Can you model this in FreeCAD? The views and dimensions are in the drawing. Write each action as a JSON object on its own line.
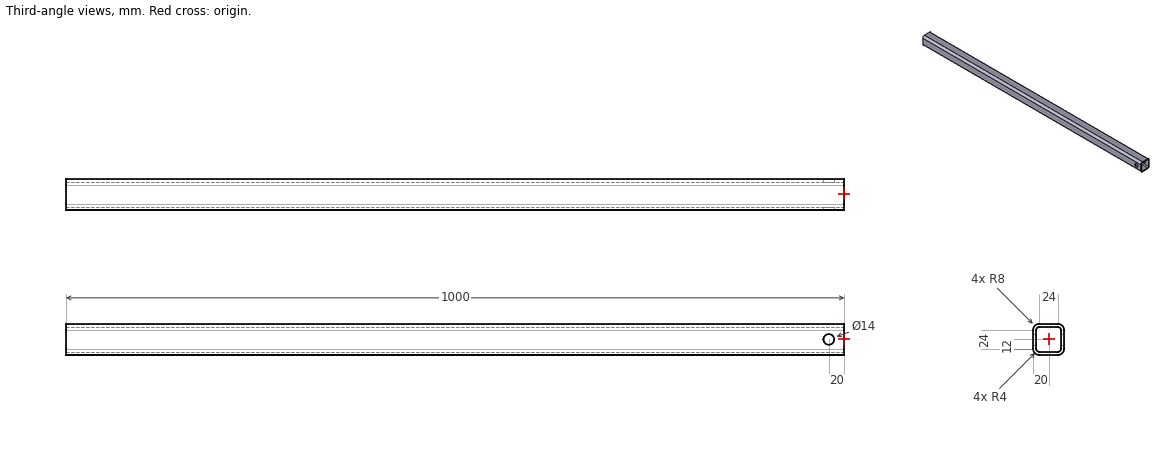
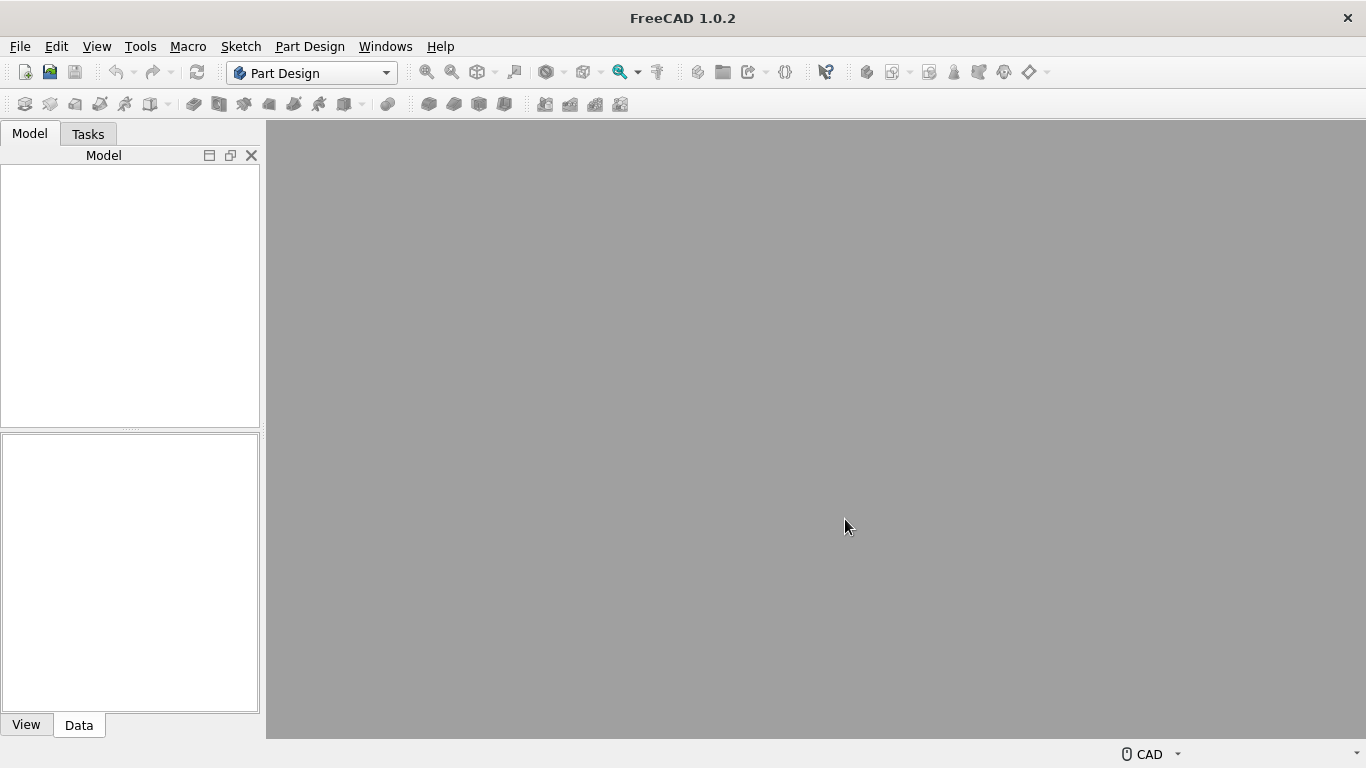
{"action": "left_click", "coordinate": [25, 72]}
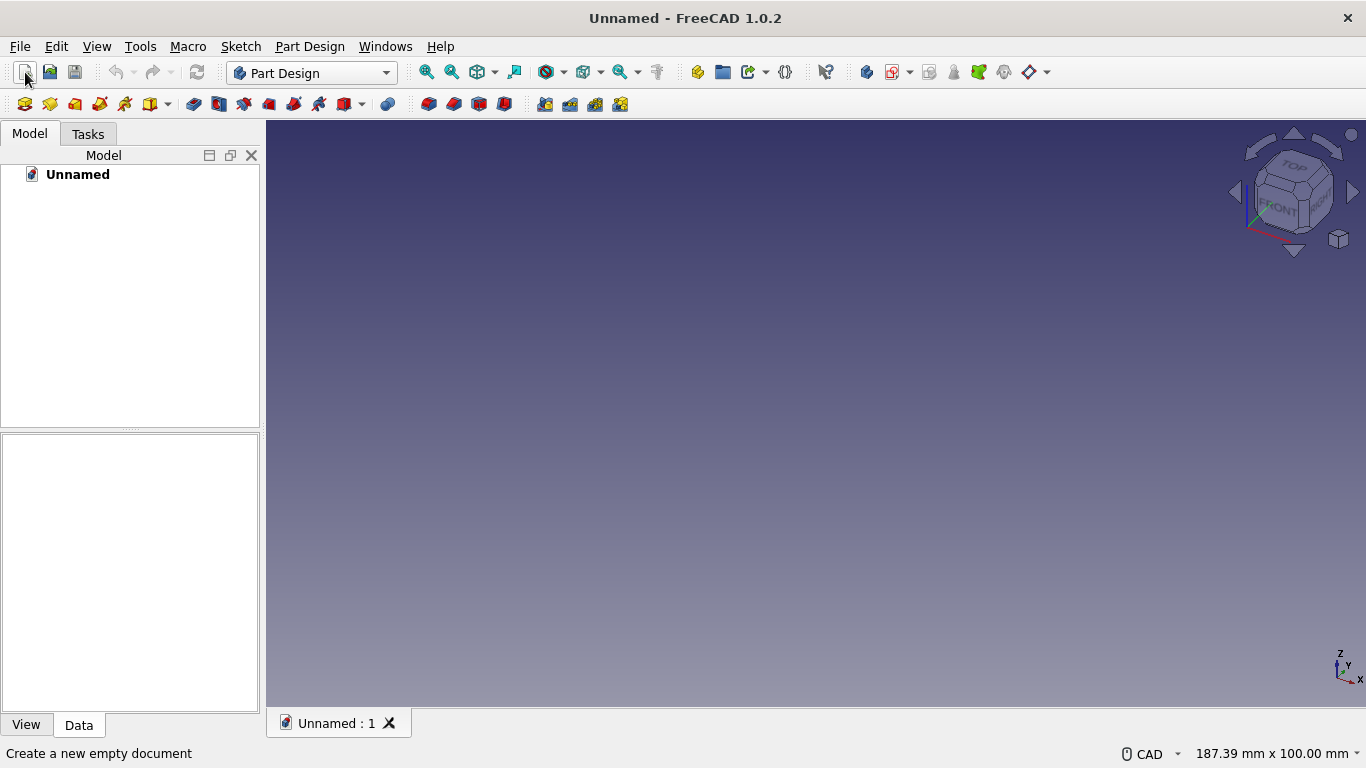
{"action": "left_click", "coordinate": [892, 72]}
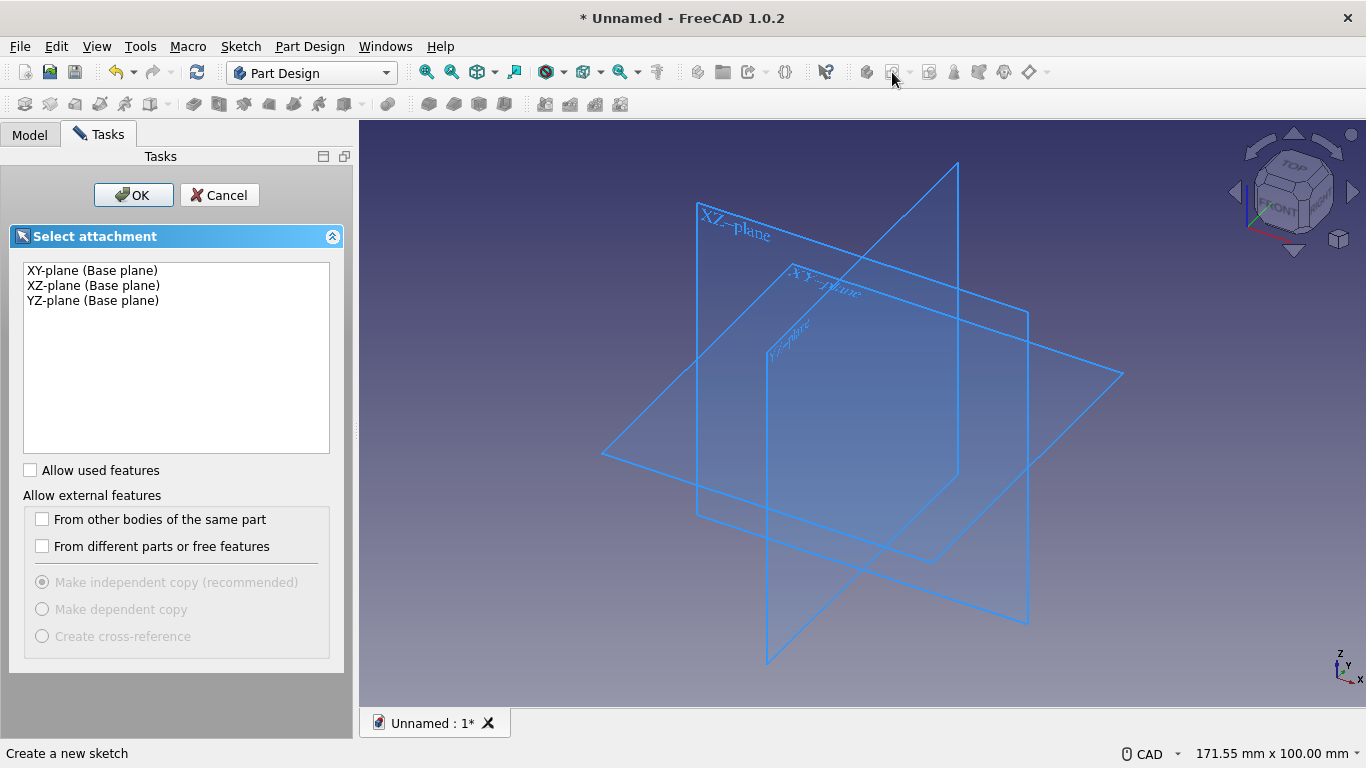
{"action": "left_click", "coordinate": [84, 300]}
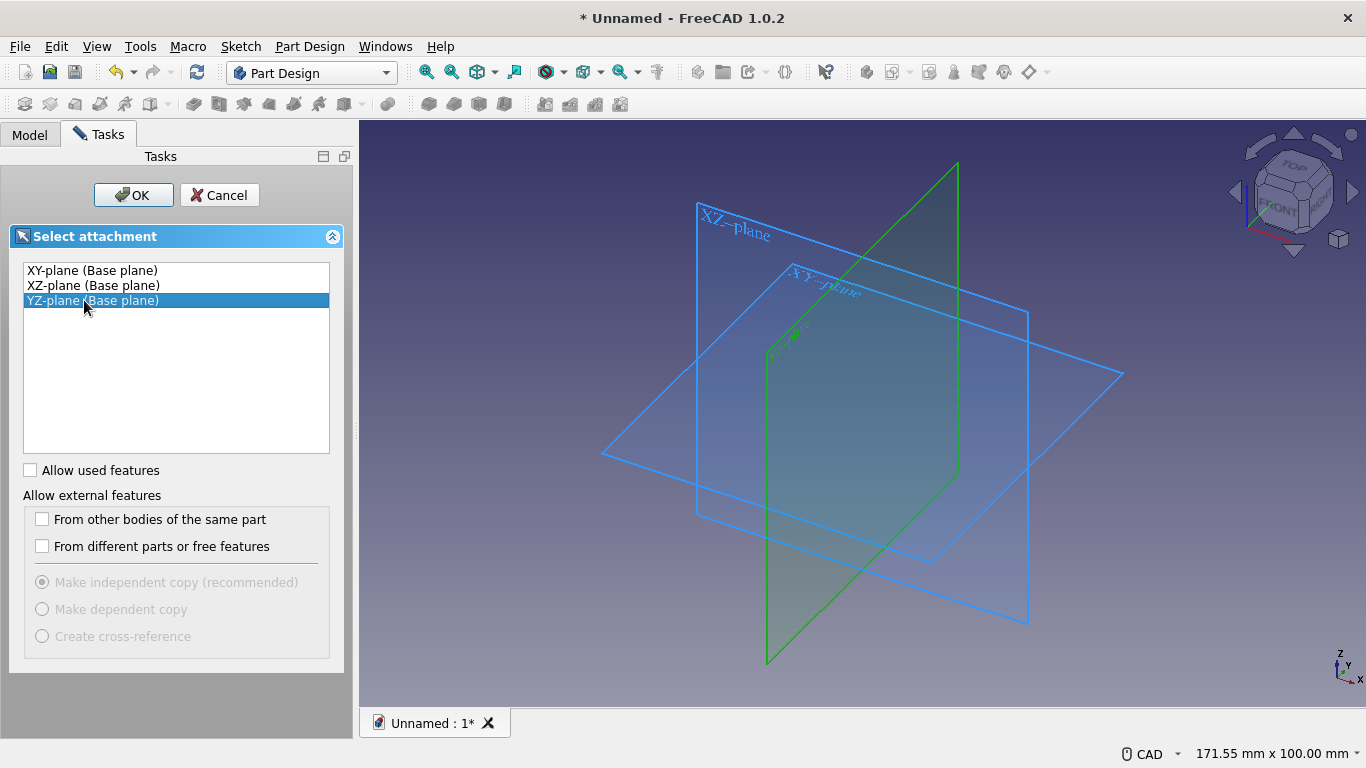
{"action": "left_click", "coordinate": [134, 195]}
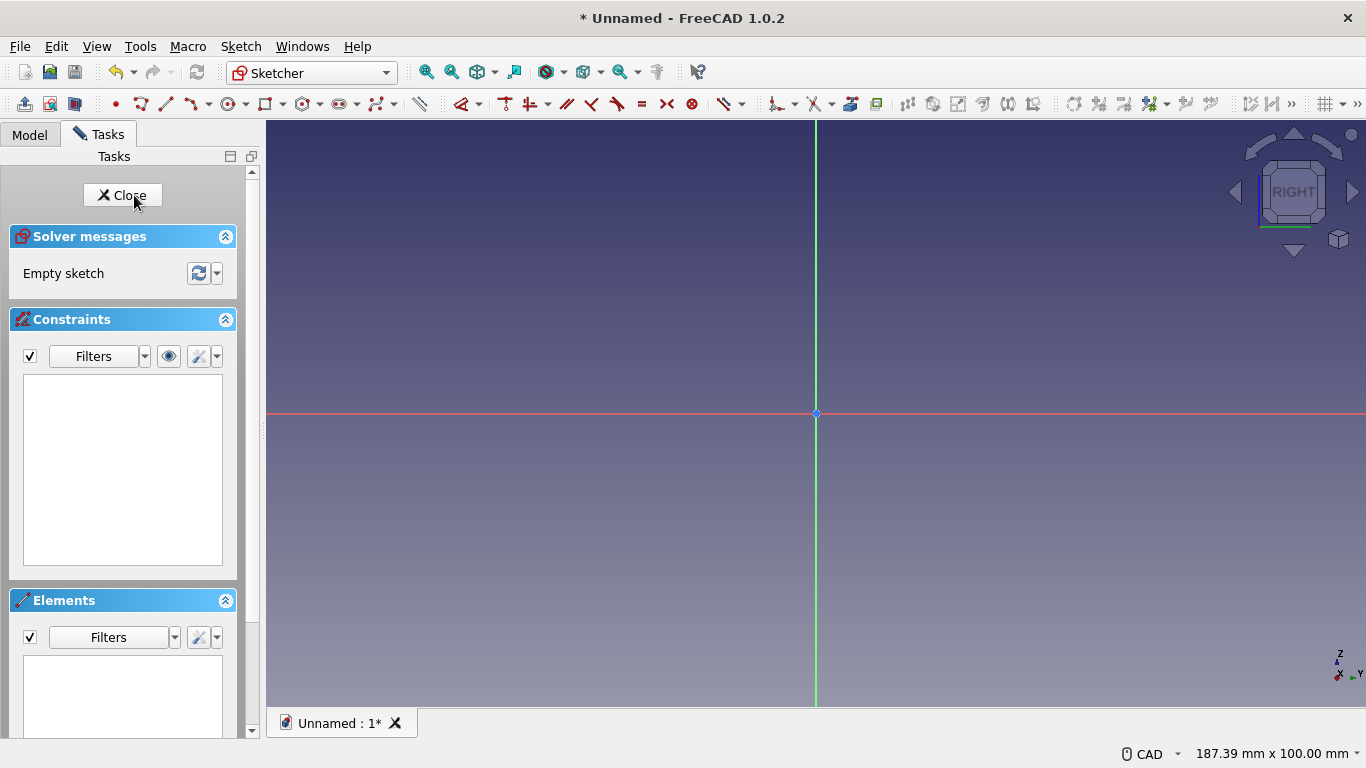
{"action": "scroll", "coordinate": [955, 413], "scroll_direction": "up", "scroll_amount": 2}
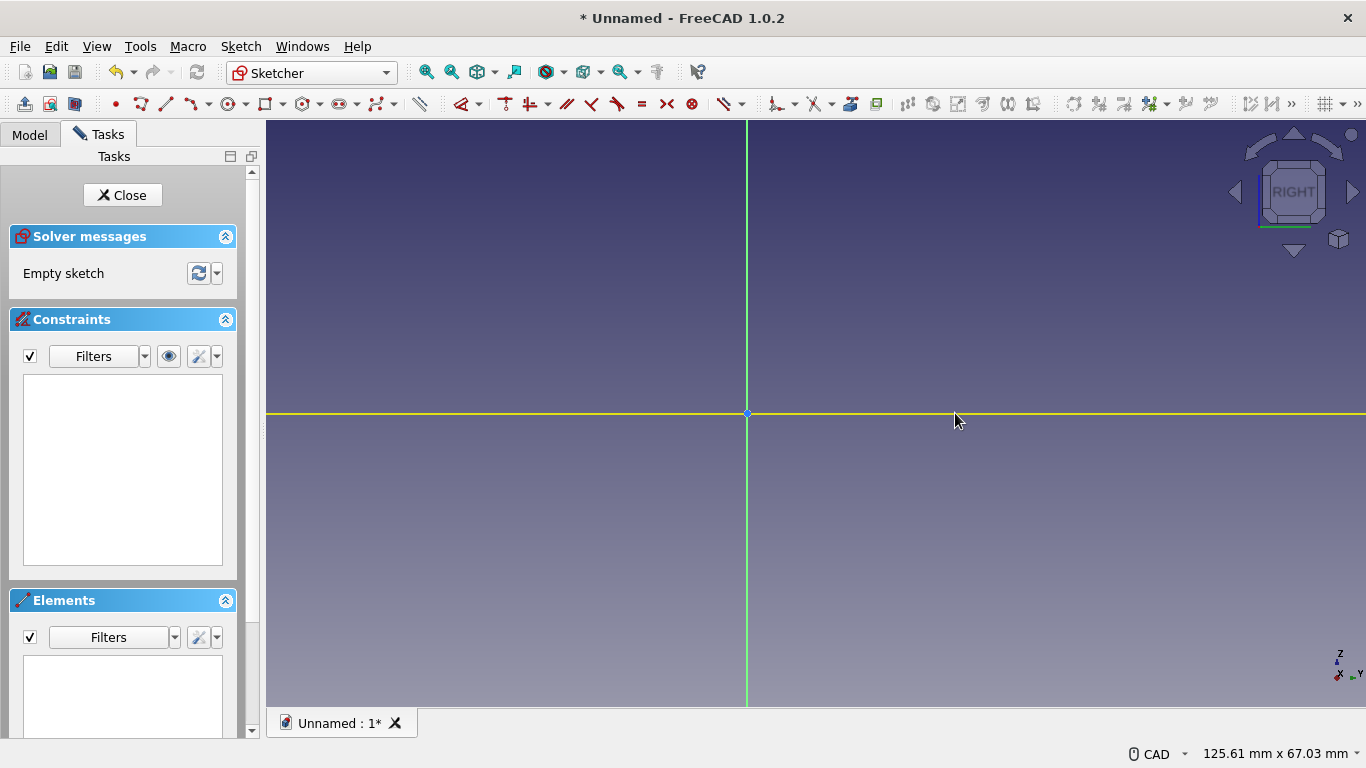
{"action": "left_click", "coordinate": [166, 104]}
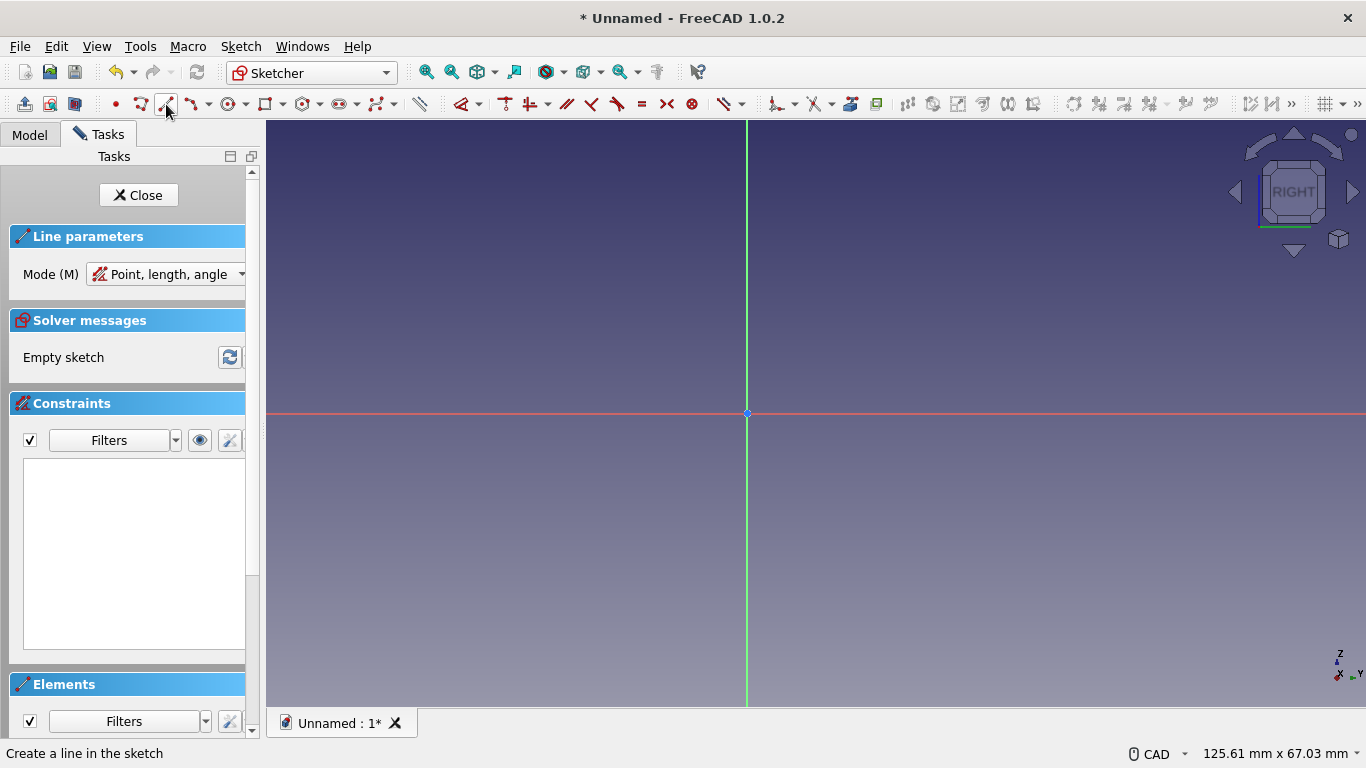
{"action": "left_click", "coordinate": [572, 519]}
{"action": "left_click", "coordinate": [572, 308]}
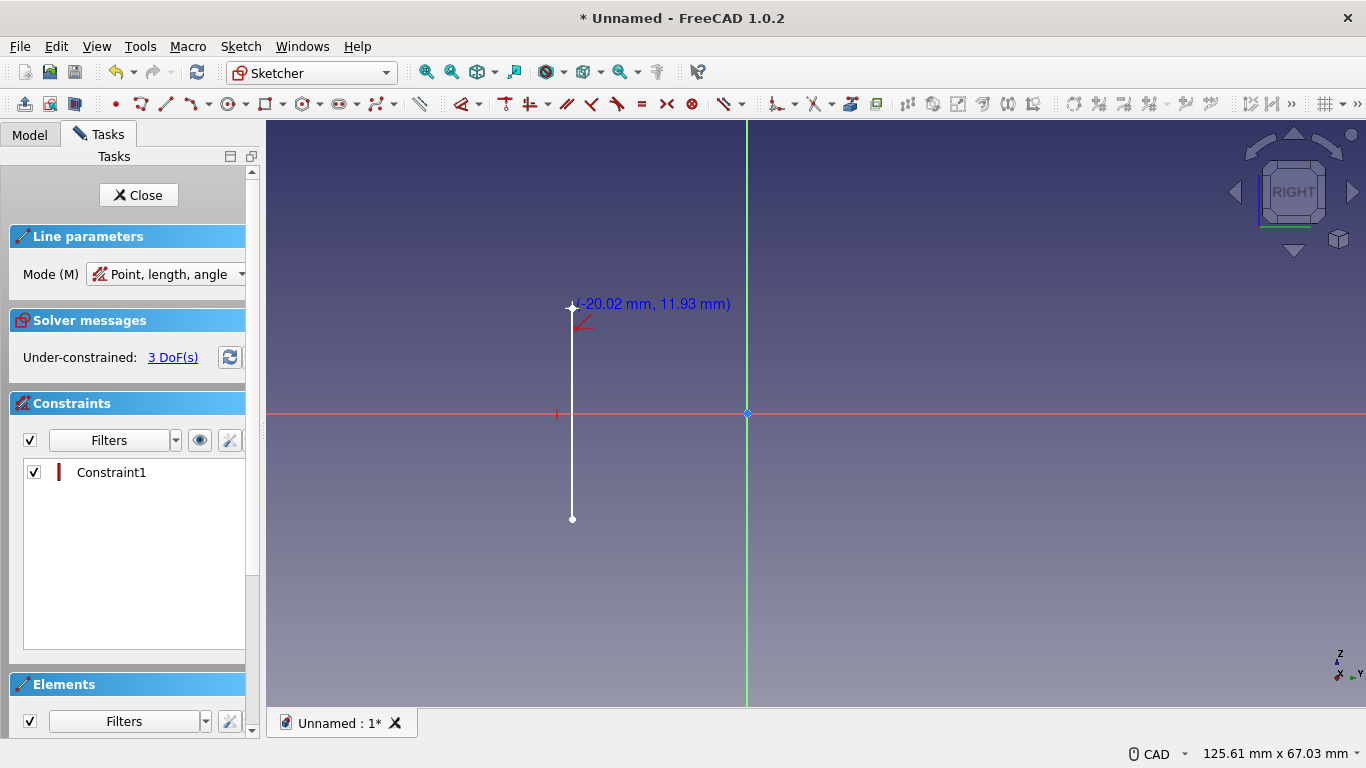
{"action": "left_click", "coordinate": [642, 238]}
{"action": "left_click", "coordinate": [852, 238]}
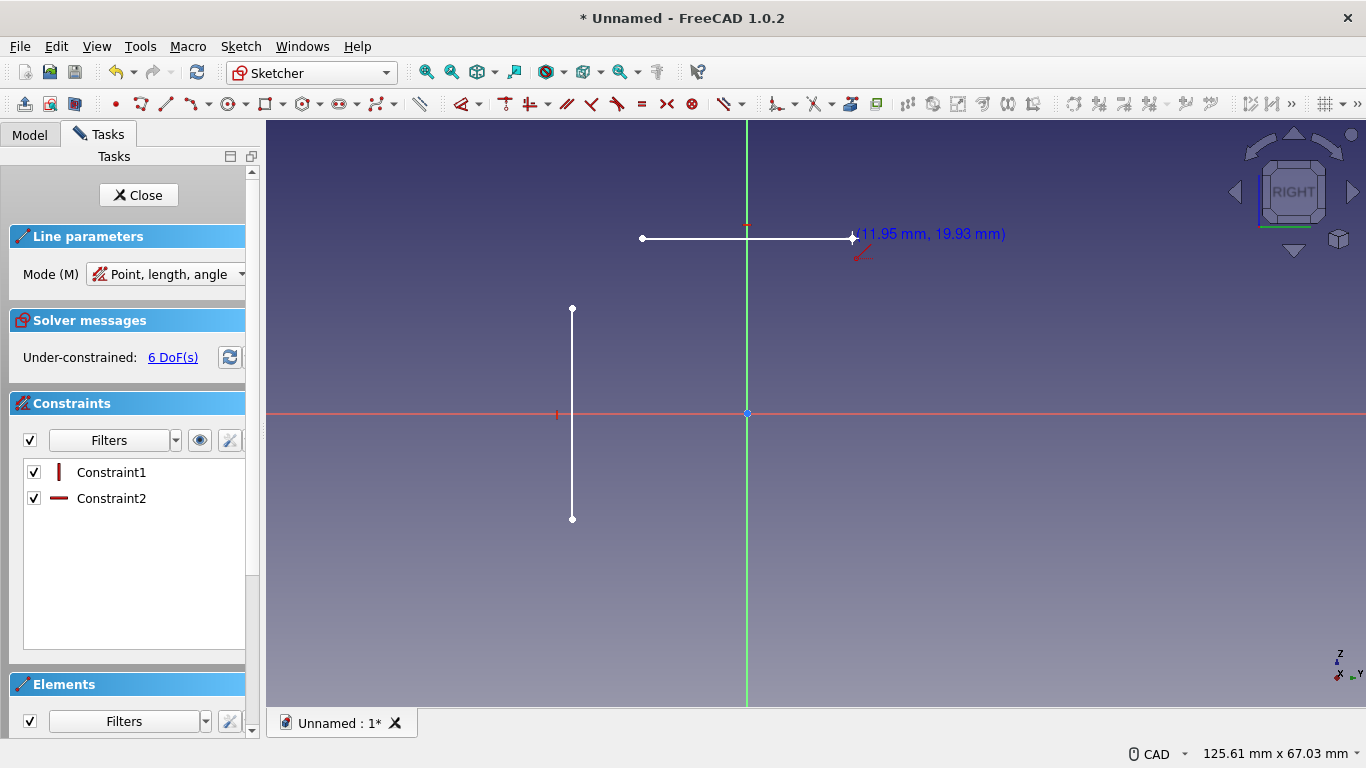
{"action": "left_click", "coordinate": [922, 308]}
{"action": "left_click", "coordinate": [922, 519]}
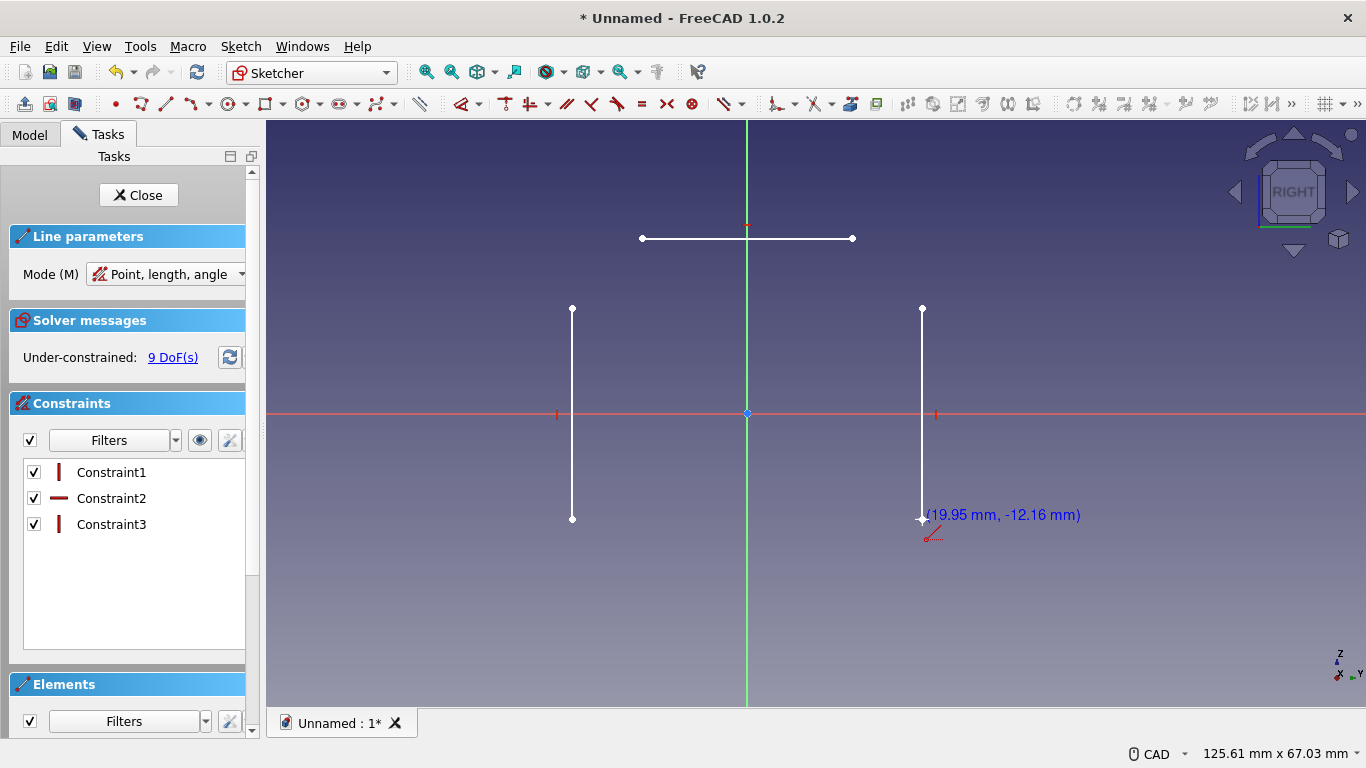
{"action": "left_click", "coordinate": [852, 589]}
{"action": "left_click", "coordinate": [642, 589]}